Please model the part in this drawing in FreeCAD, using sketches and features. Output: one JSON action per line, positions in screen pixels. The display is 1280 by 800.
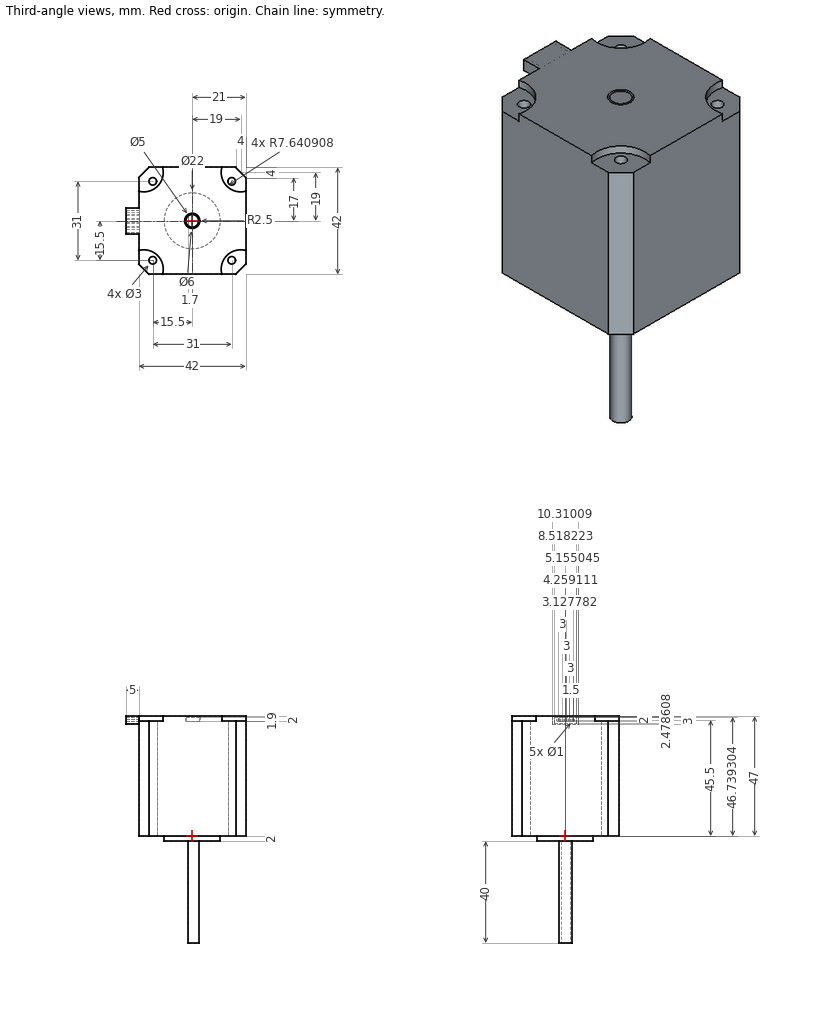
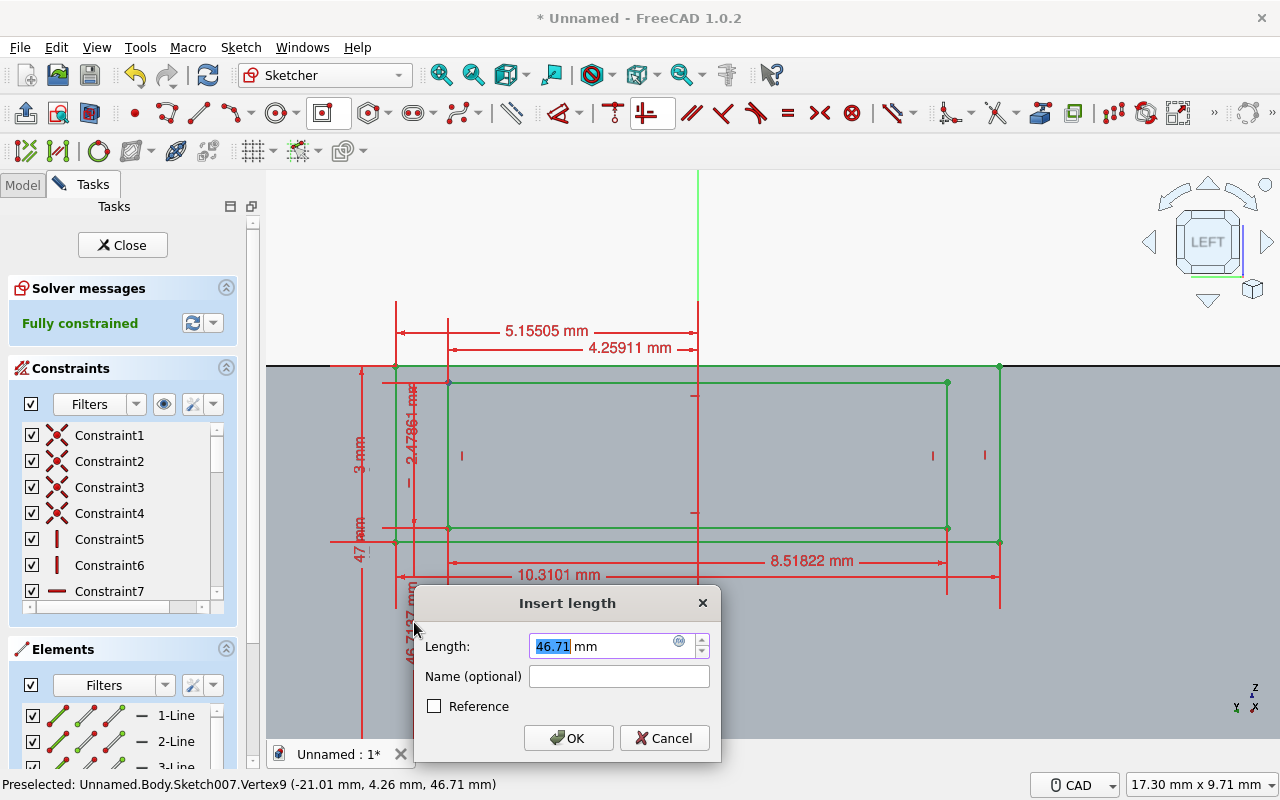
{"action": "type", "text": "46.739304"}
{"action": "key", "text": "Return"}
{"action": "key", "text": "Escape"}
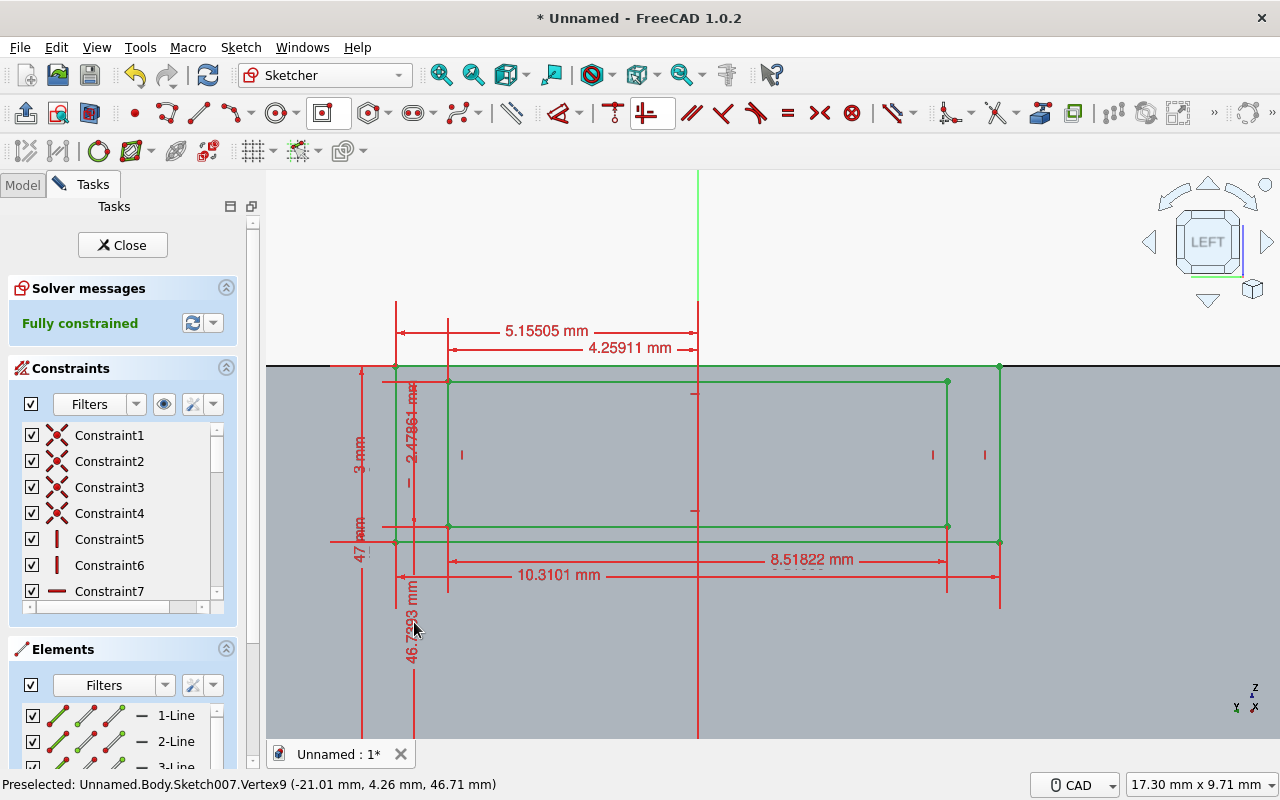
{"action": "left_click", "coordinate": [123, 245]}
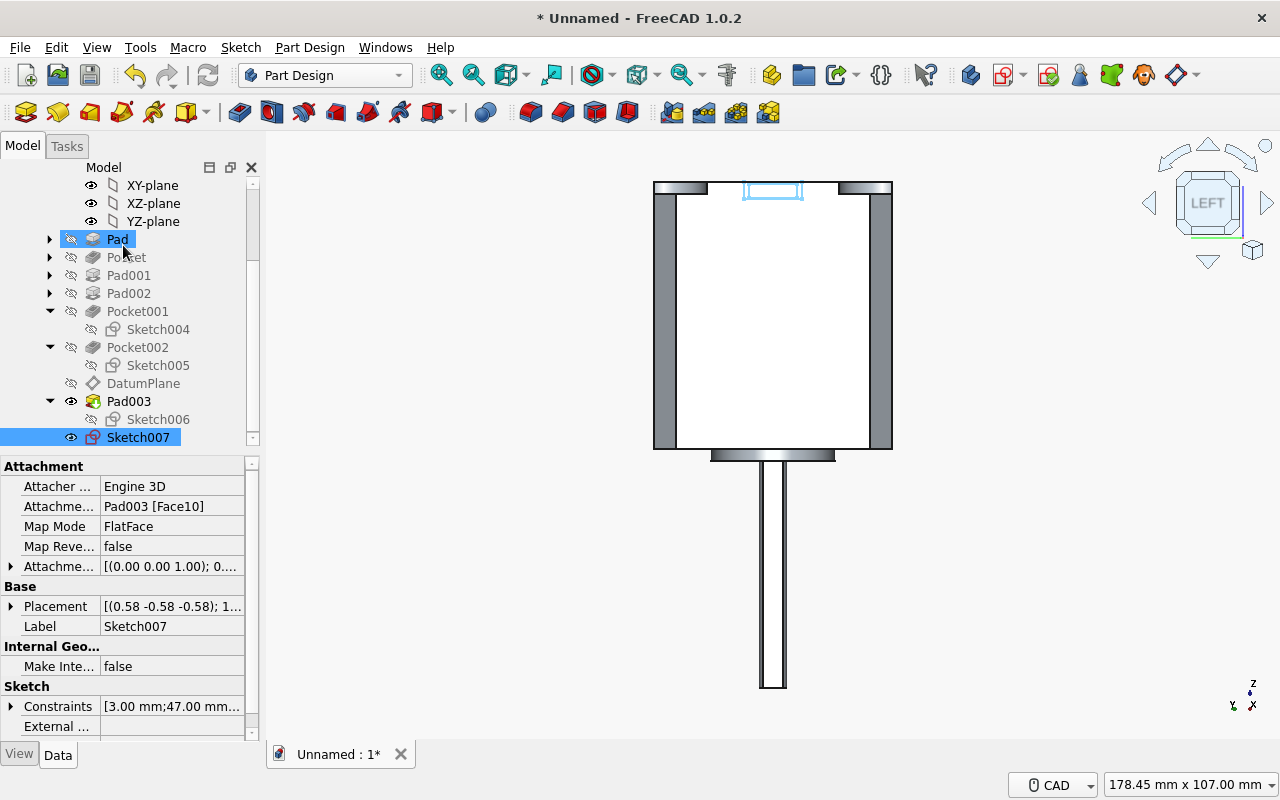
{"action": "left_click", "coordinate": [26, 112]}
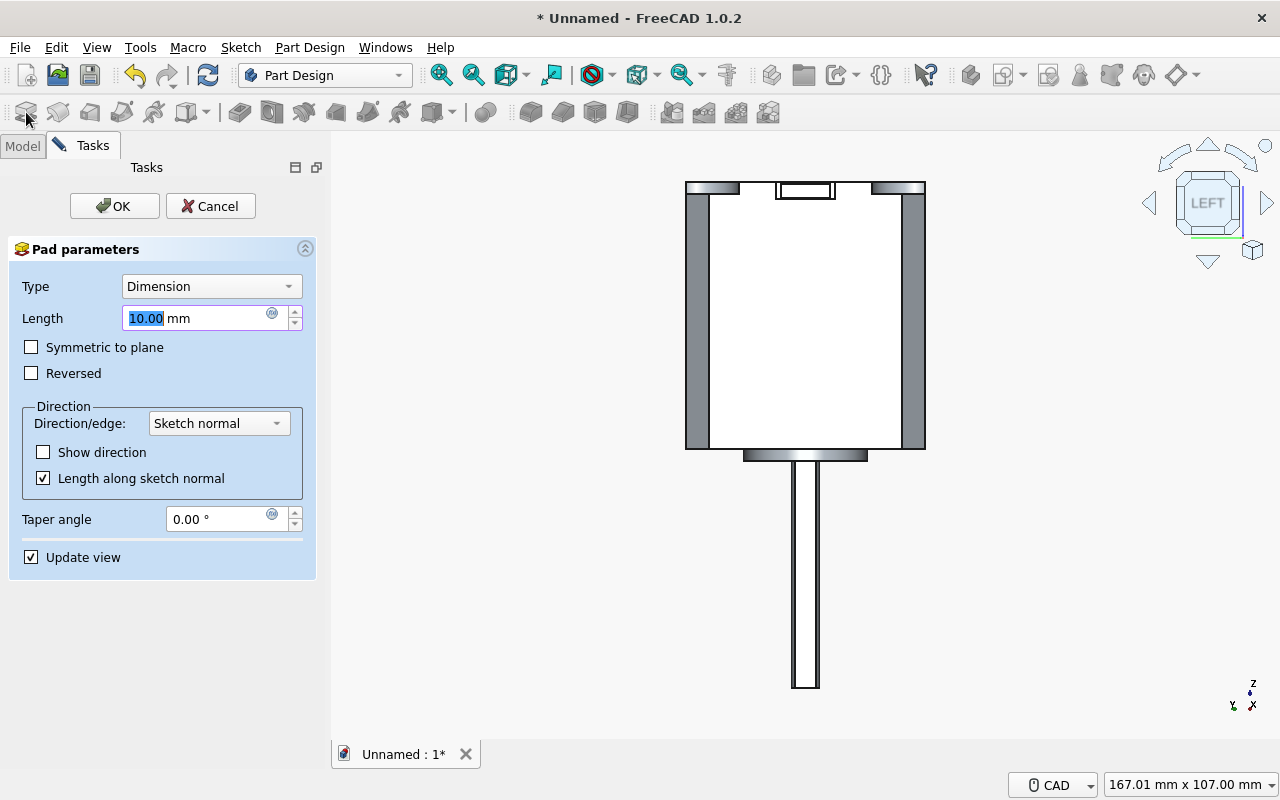
{"action": "type", "text": "5"}
{"action": "key", "text": "Tab"}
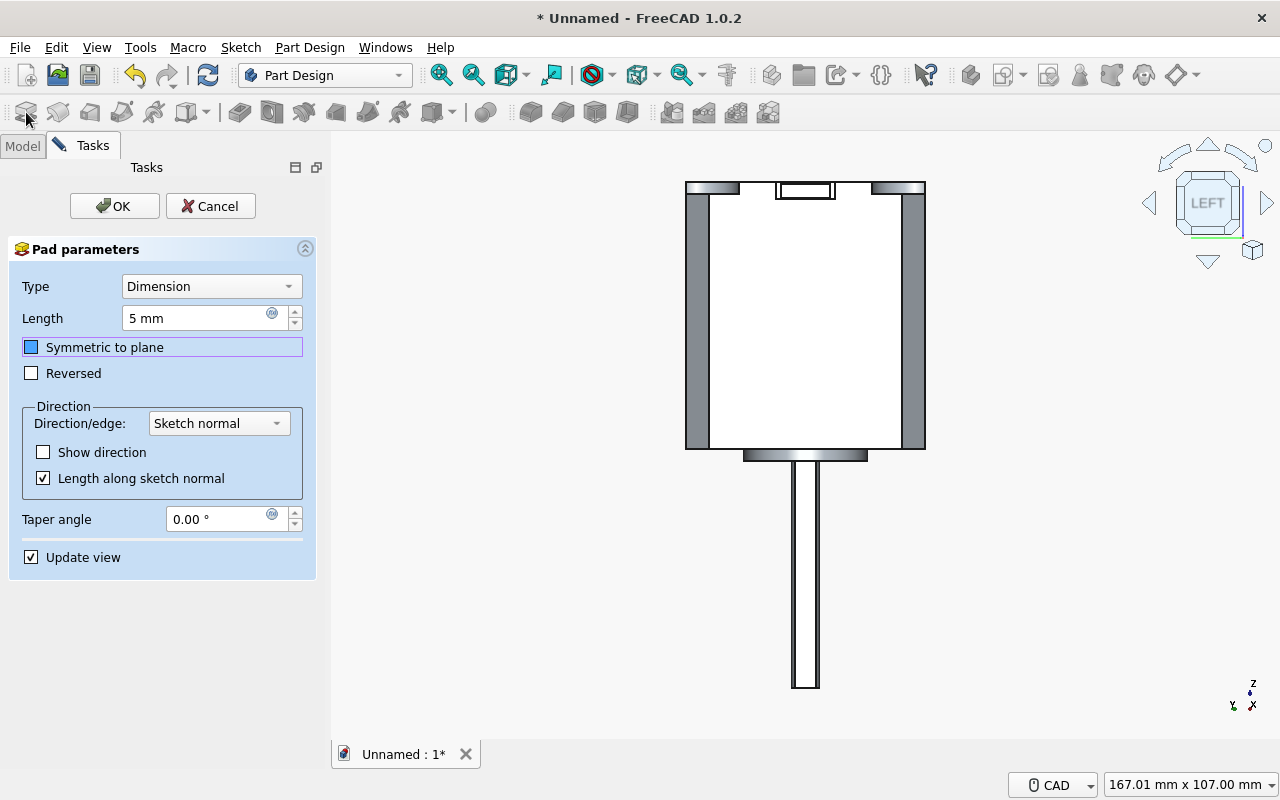
{"action": "left_click", "coordinate": [115, 206]}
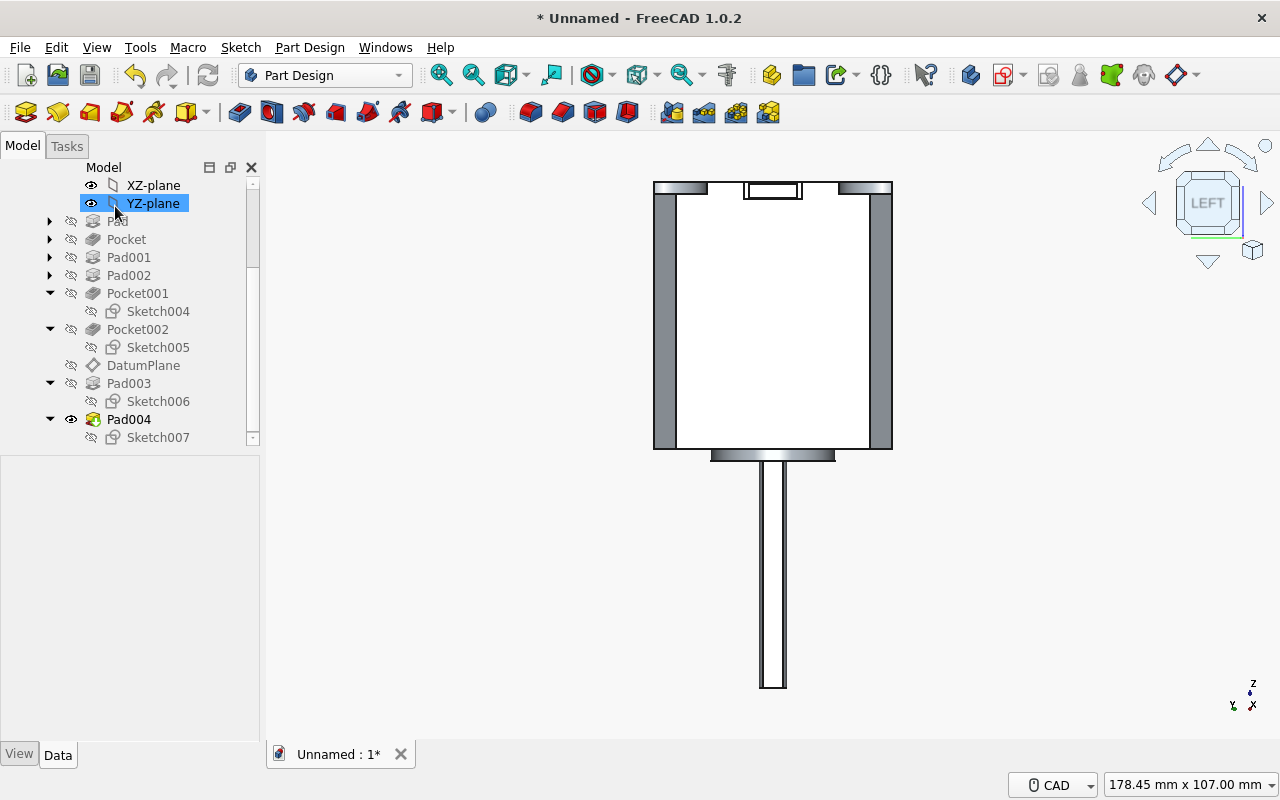
{"action": "left_click", "coordinate": [773, 315]}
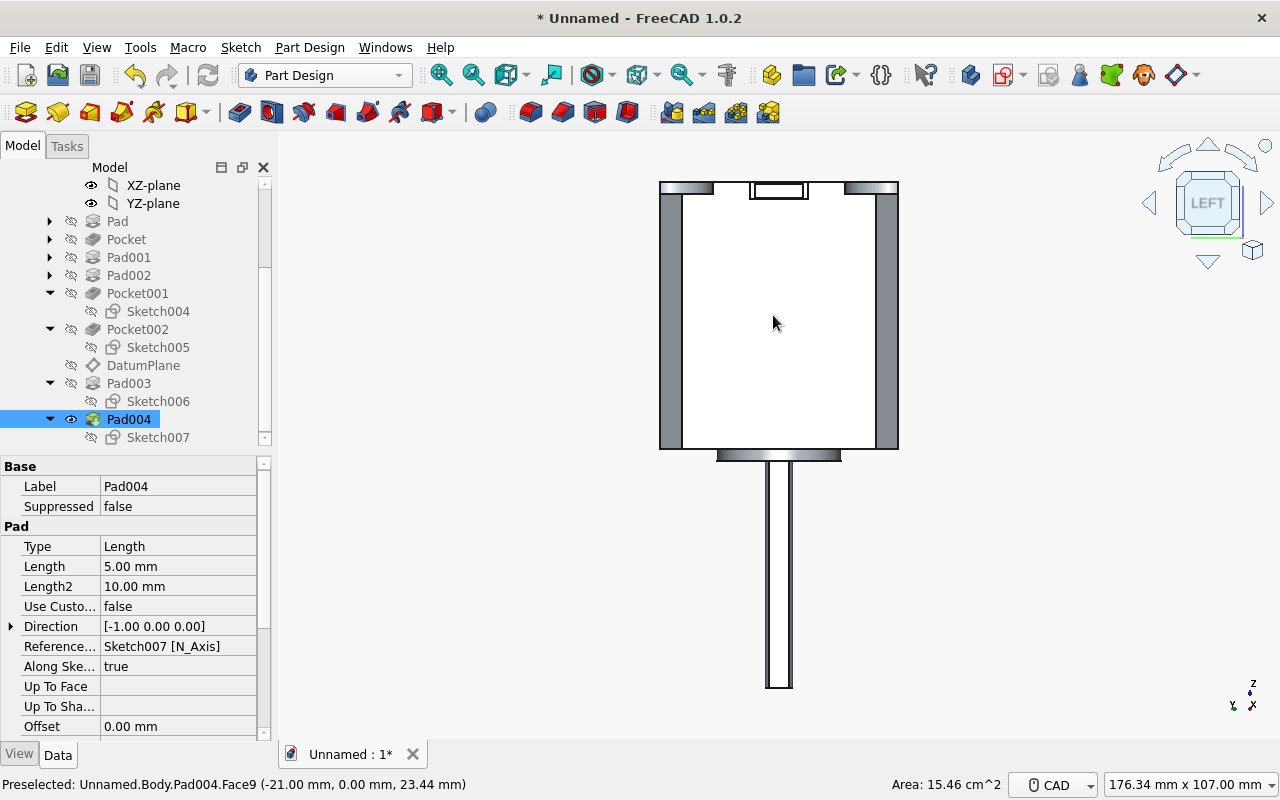
{"action": "left_click", "coordinate": [1004, 76]}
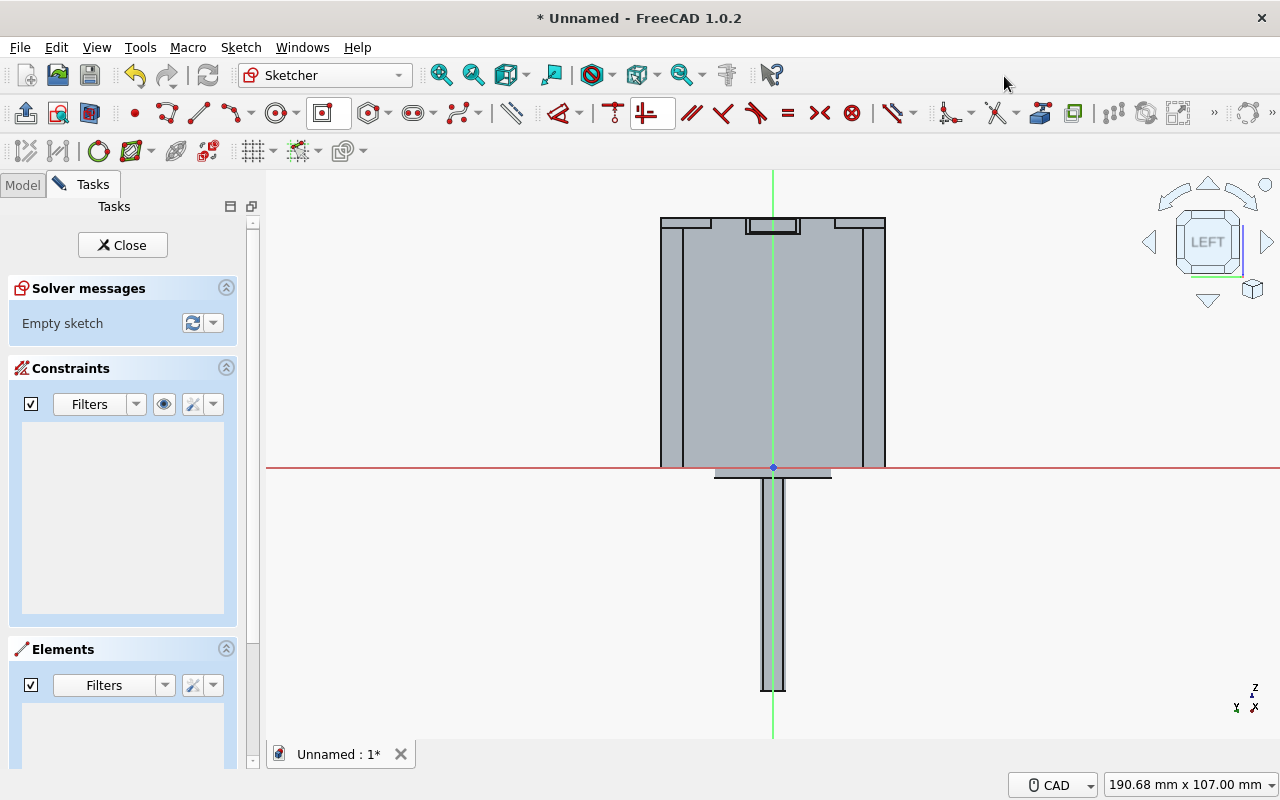
{"action": "scroll", "coordinate": [777, 211], "scroll_direction": "up", "scroll_amount": 14}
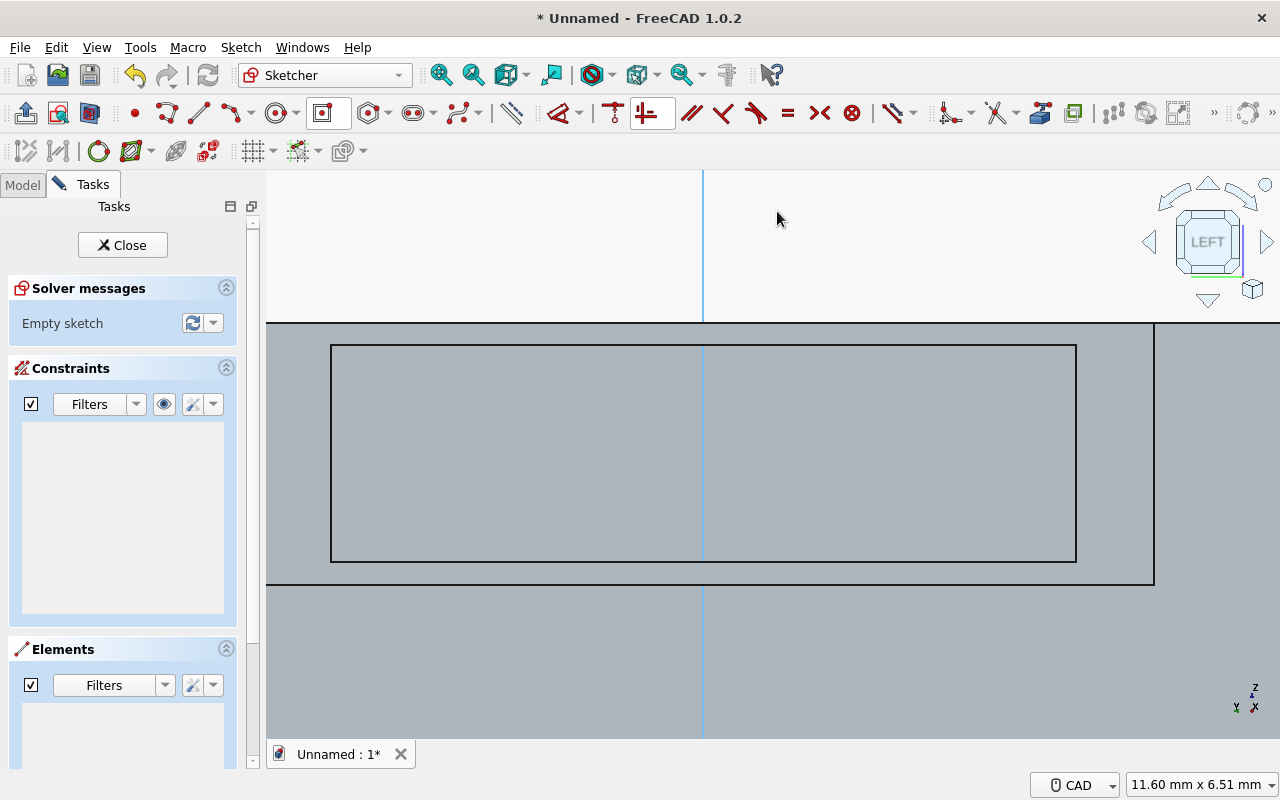
{"action": "left_click", "coordinate": [276, 114]}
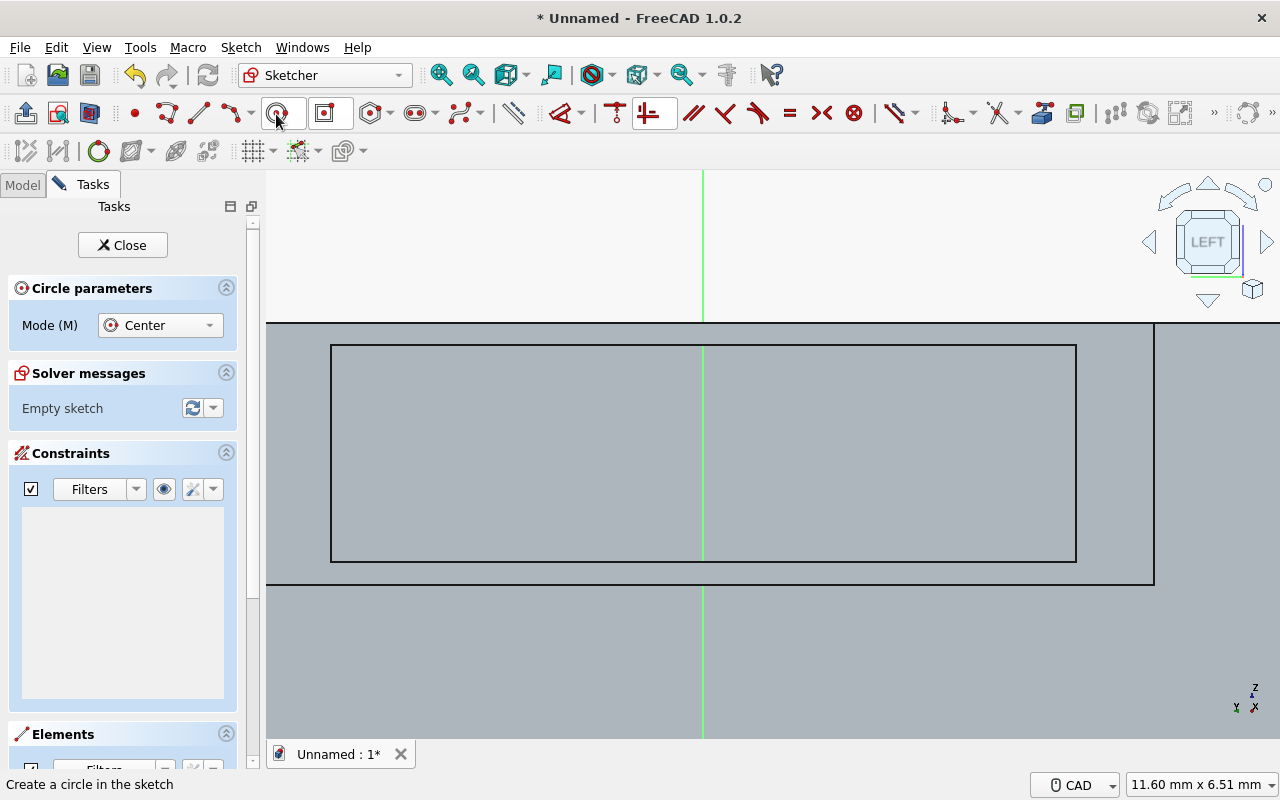
{"action": "left_click", "coordinate": [430, 454]}
{"action": "left_click", "coordinate": [461, 423]}